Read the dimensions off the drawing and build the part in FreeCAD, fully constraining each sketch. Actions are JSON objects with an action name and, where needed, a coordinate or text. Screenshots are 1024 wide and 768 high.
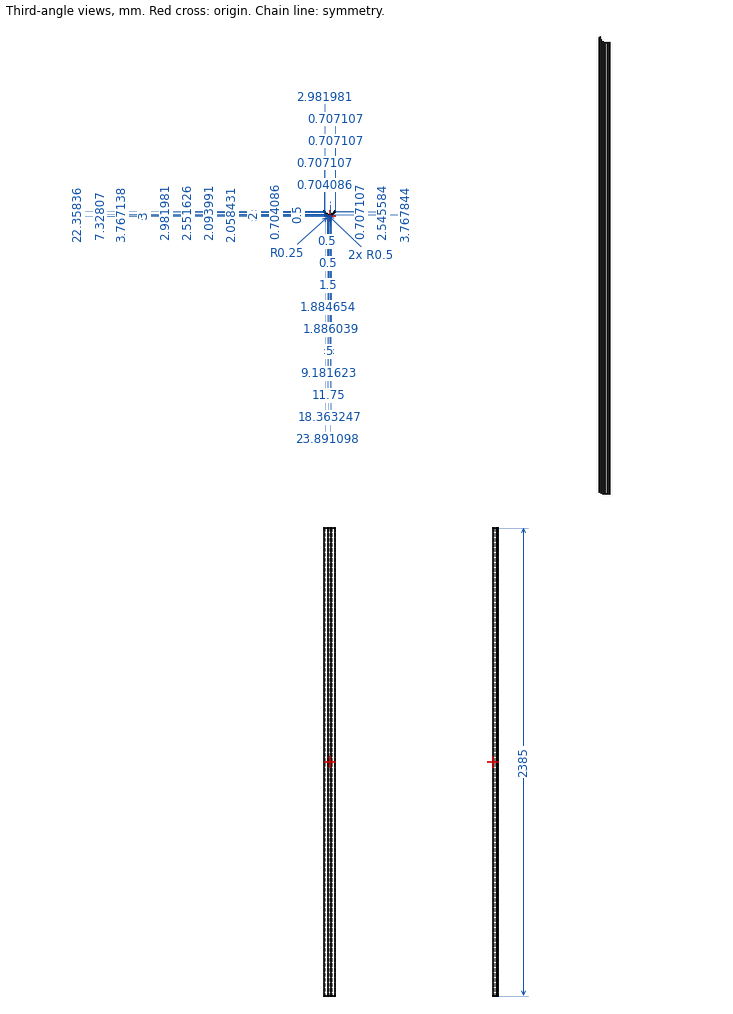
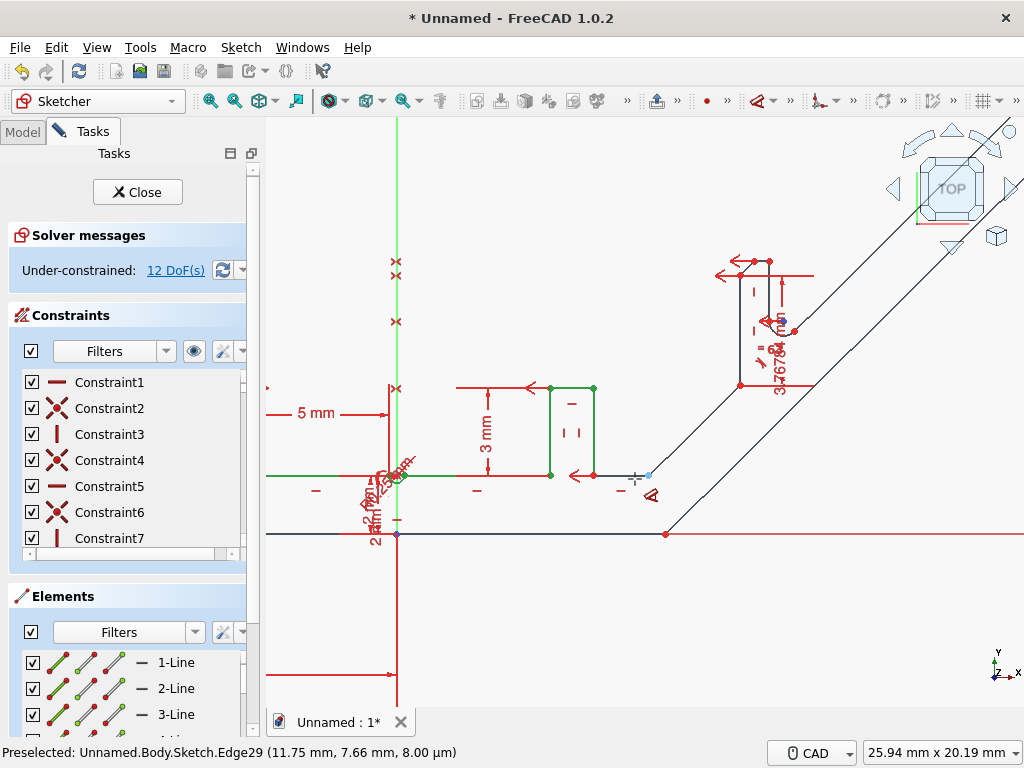
{"action": "left_click", "coordinate": [632, 476]}
{"action": "left_click", "coordinate": [621, 510]}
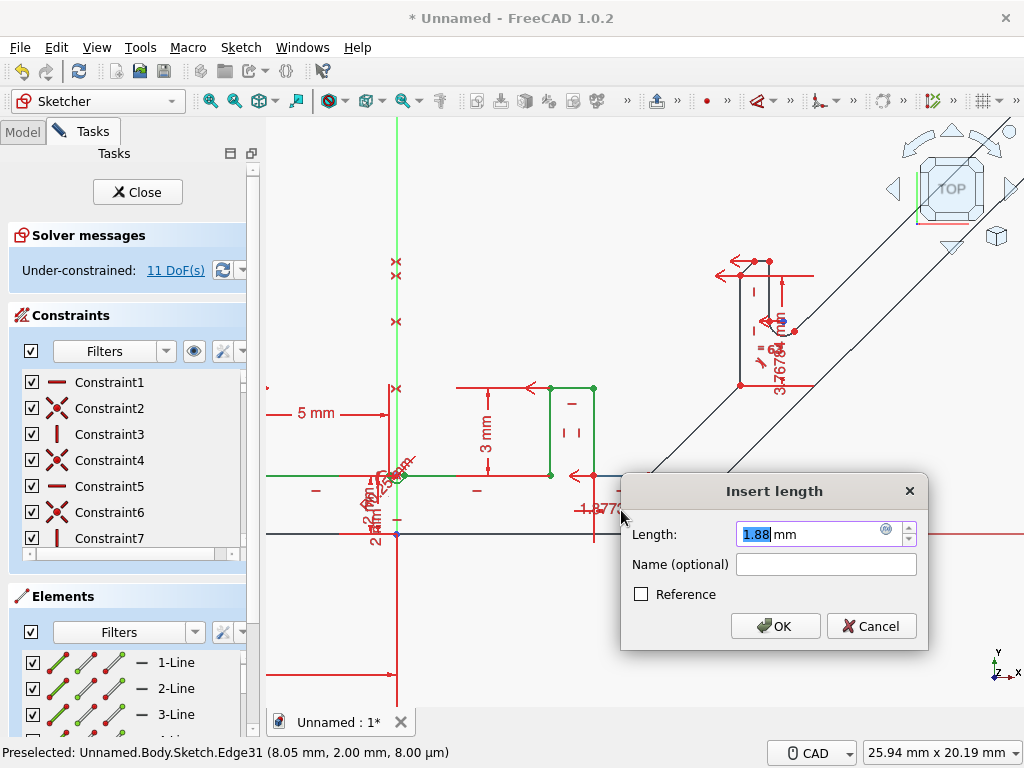
{"action": "type", "text": "1.886039"}
{"action": "key", "text": "Return"}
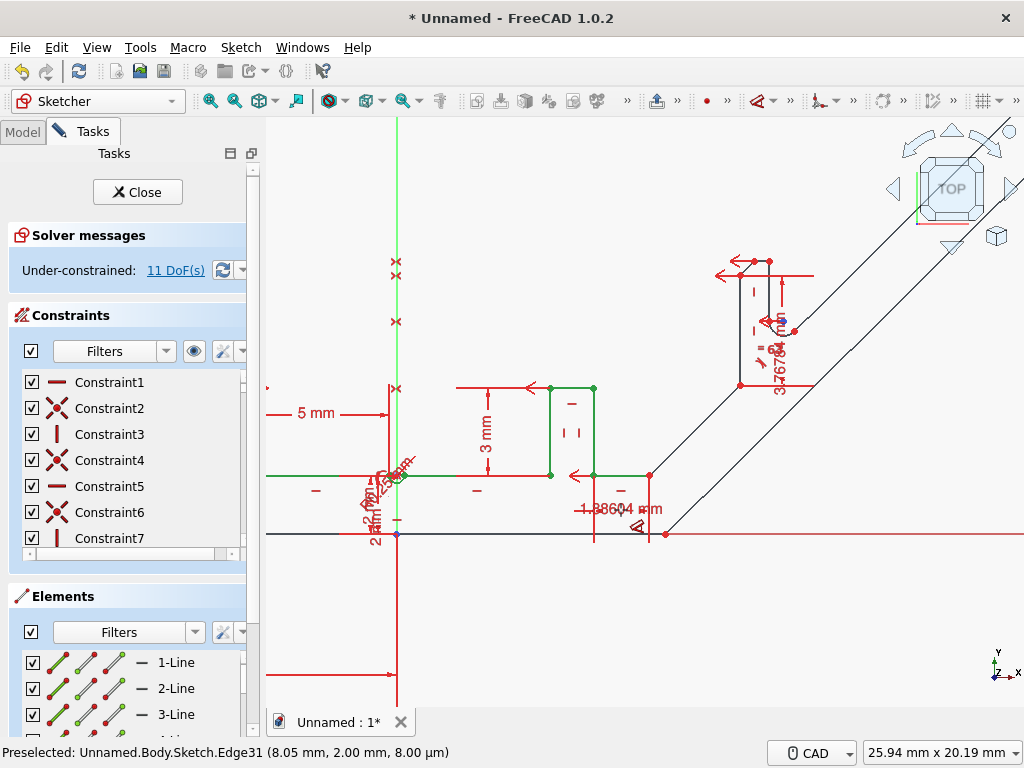
{"action": "scroll", "coordinate": [635, 479], "scroll_direction": "down", "scroll_amount": 7}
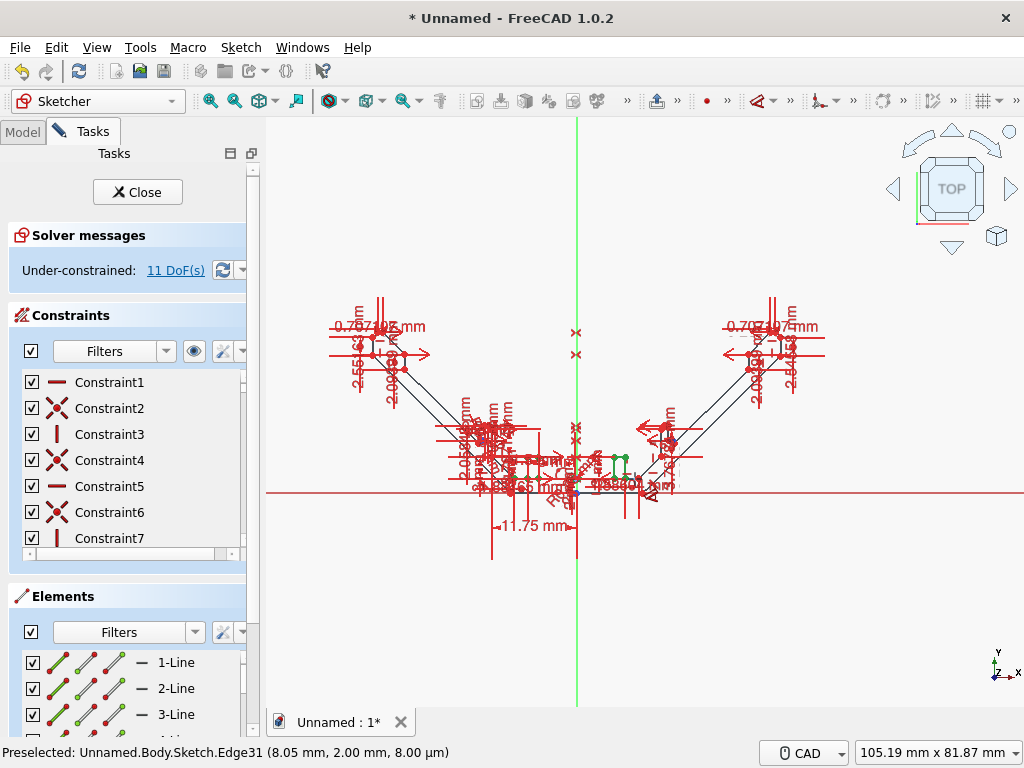
{"action": "scroll", "coordinate": [485, 441], "scroll_direction": "up", "scroll_amount": 7}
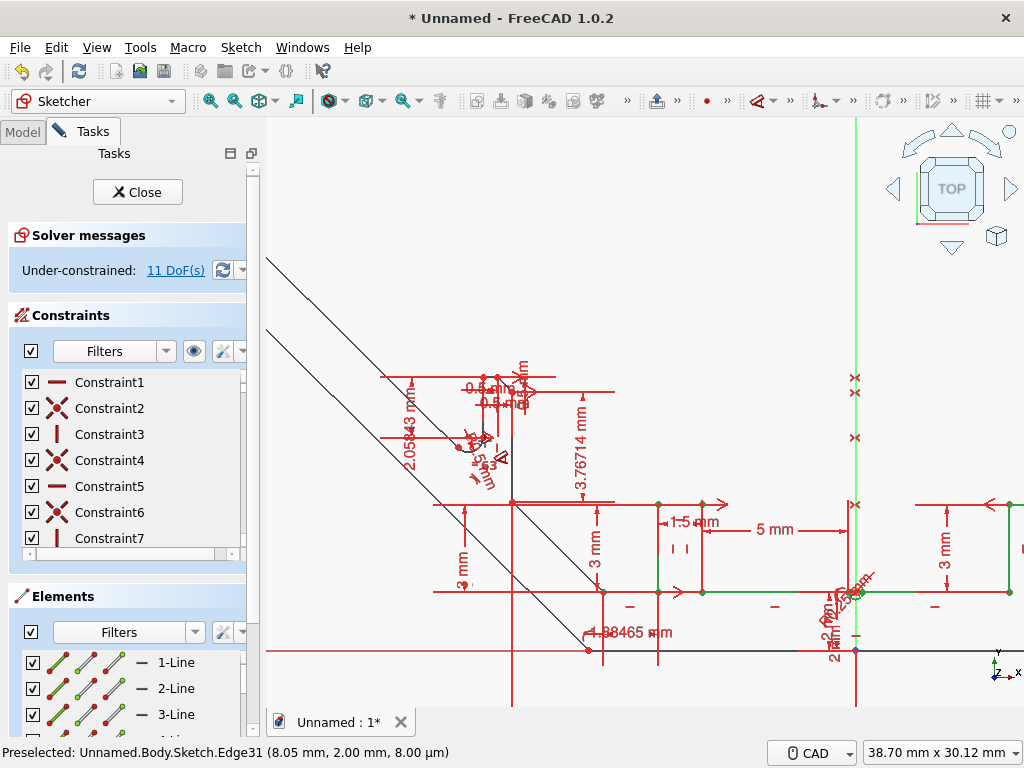
{"action": "left_click", "coordinate": [483, 438]}
{"action": "left_click", "coordinate": [449, 544]}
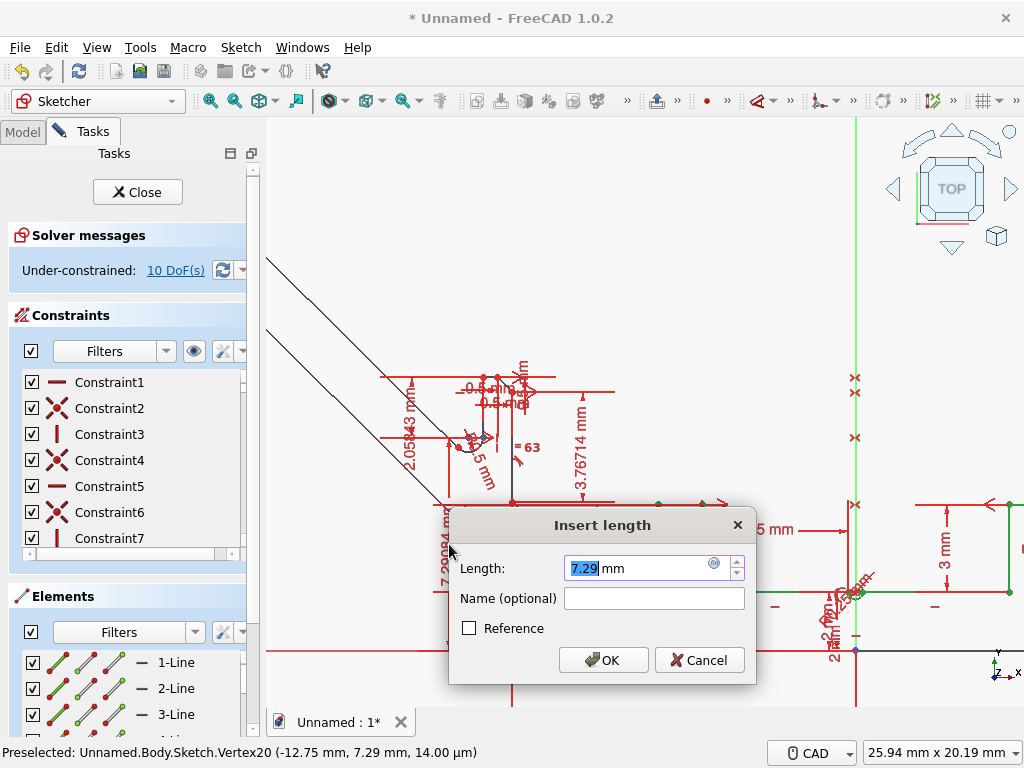
{"action": "type", "text": "7.32807"}
{"action": "key", "text": "Return"}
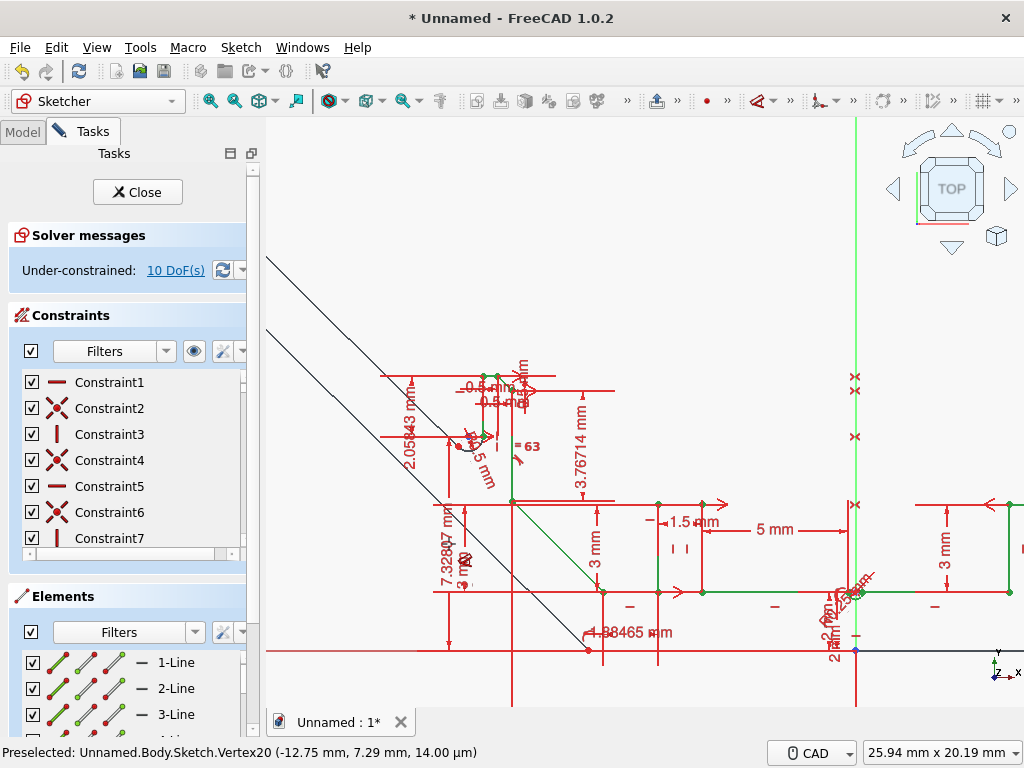
{"action": "scroll", "coordinate": [485, 441], "scroll_direction": "down", "scroll_amount": 7}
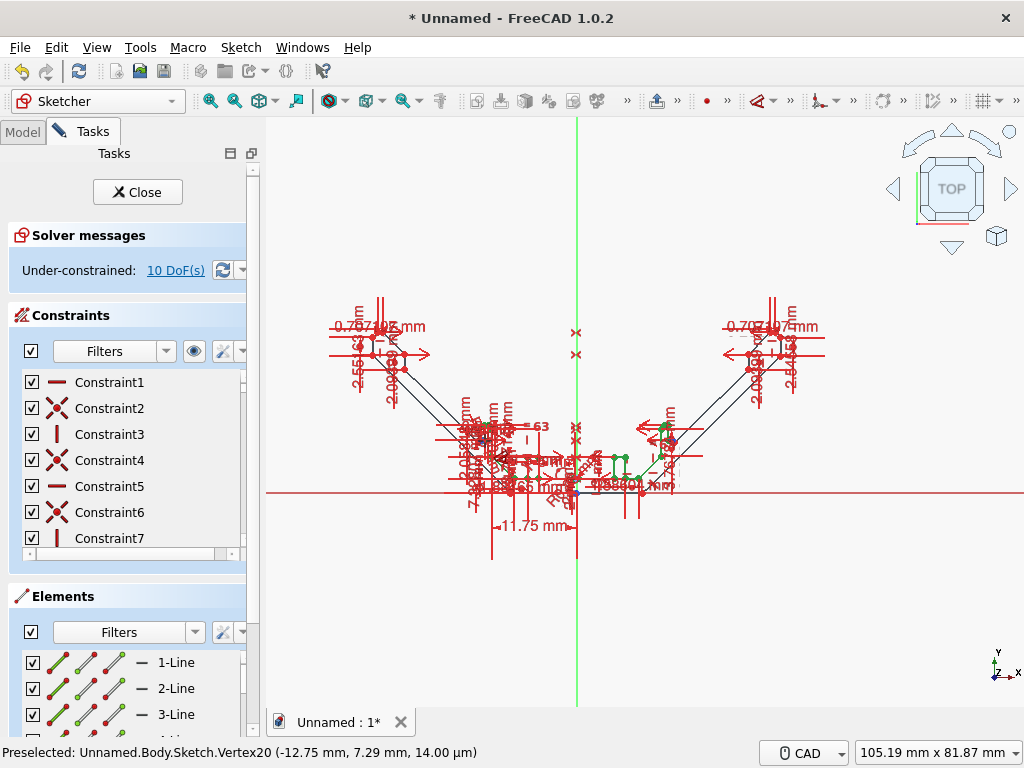
{"action": "left_click", "coordinate": [550, 493]}
{"action": "left_click", "coordinate": [607, 527]}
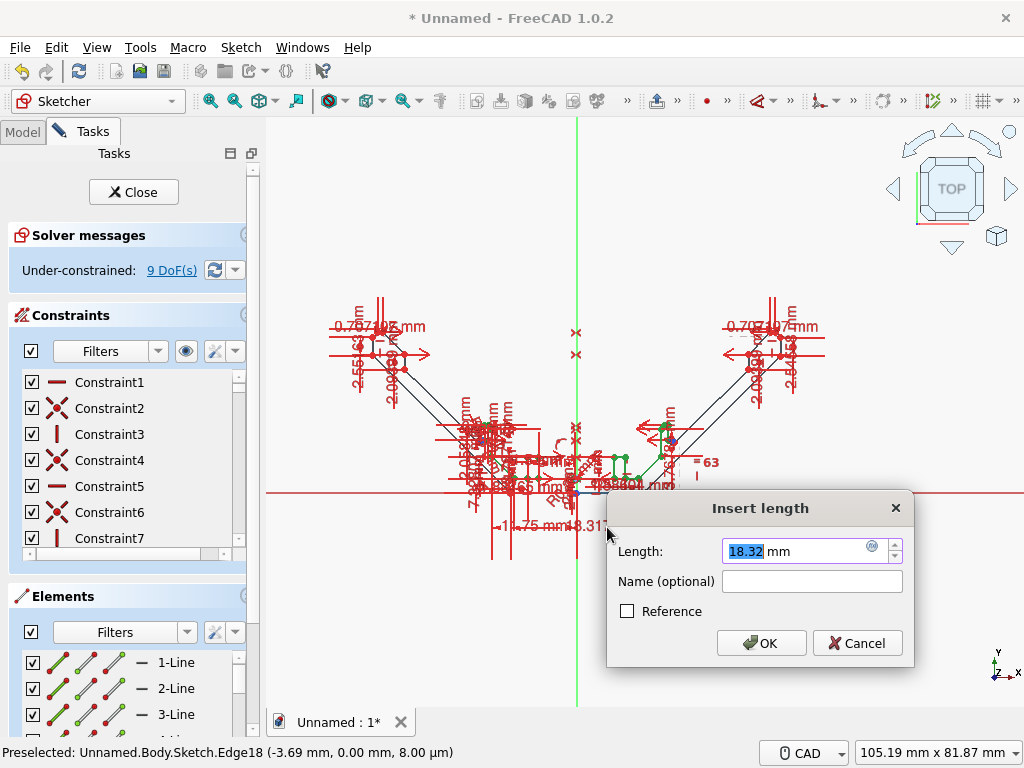
{"action": "type", "text": "18.363247"}
{"action": "key", "text": "Return"}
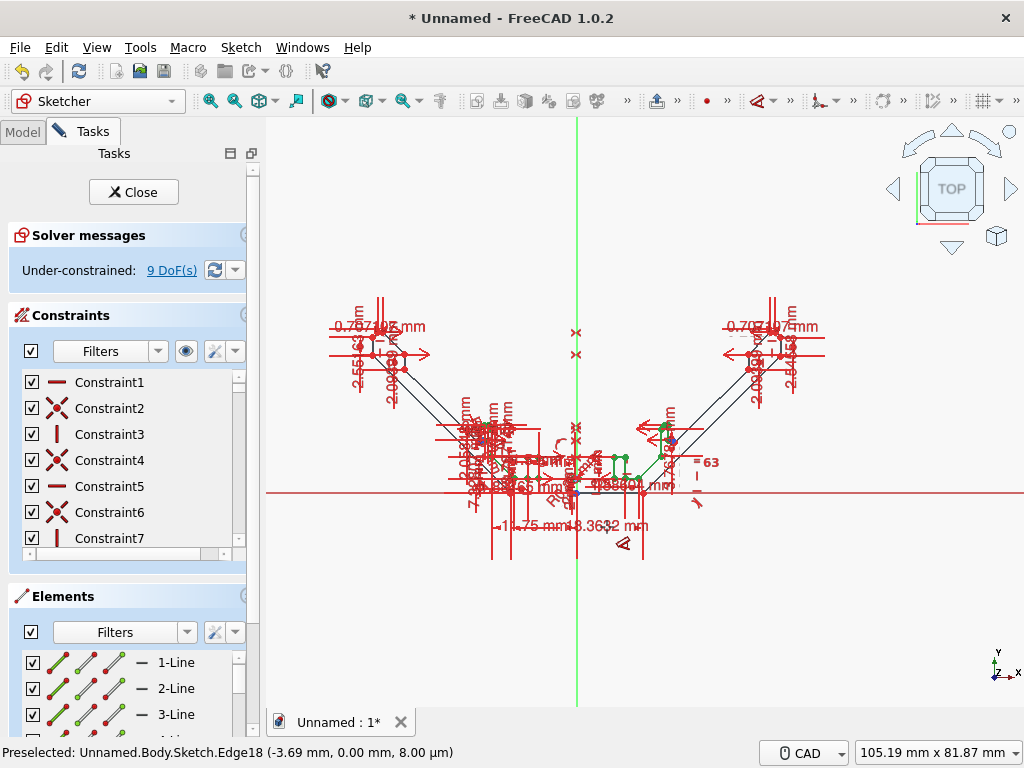
{"action": "scroll", "coordinate": [383, 332], "scroll_direction": "up", "scroll_amount": 5}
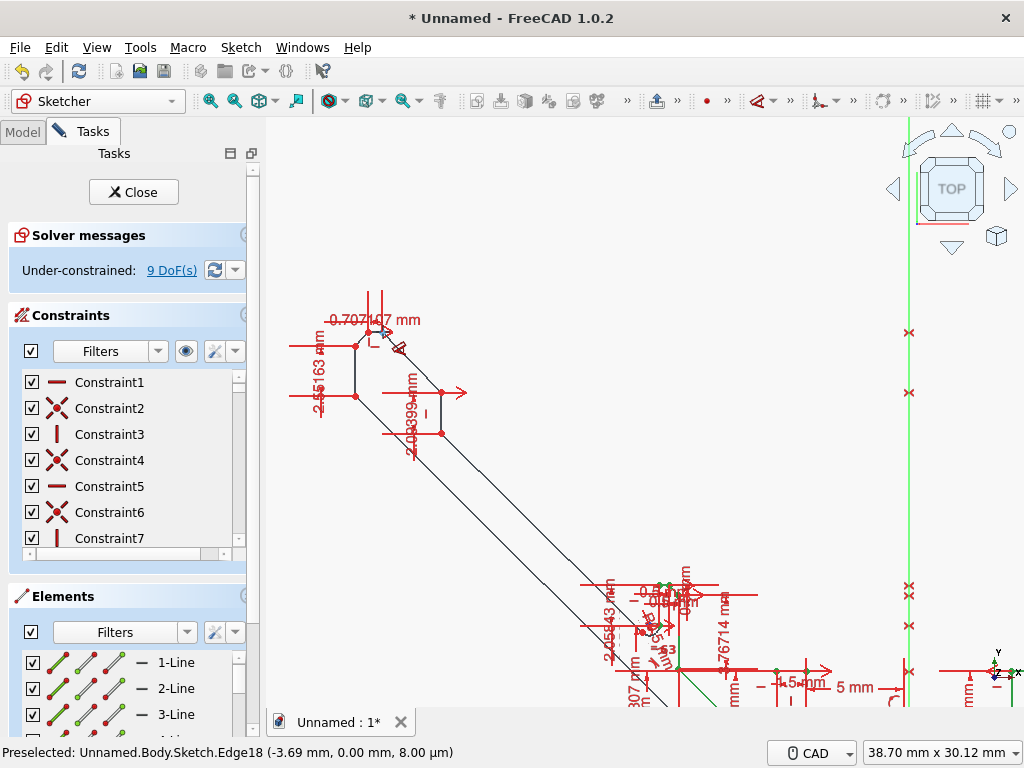
{"action": "left_click", "coordinate": [382, 332]}
{"action": "left_click", "coordinate": [348, 506]}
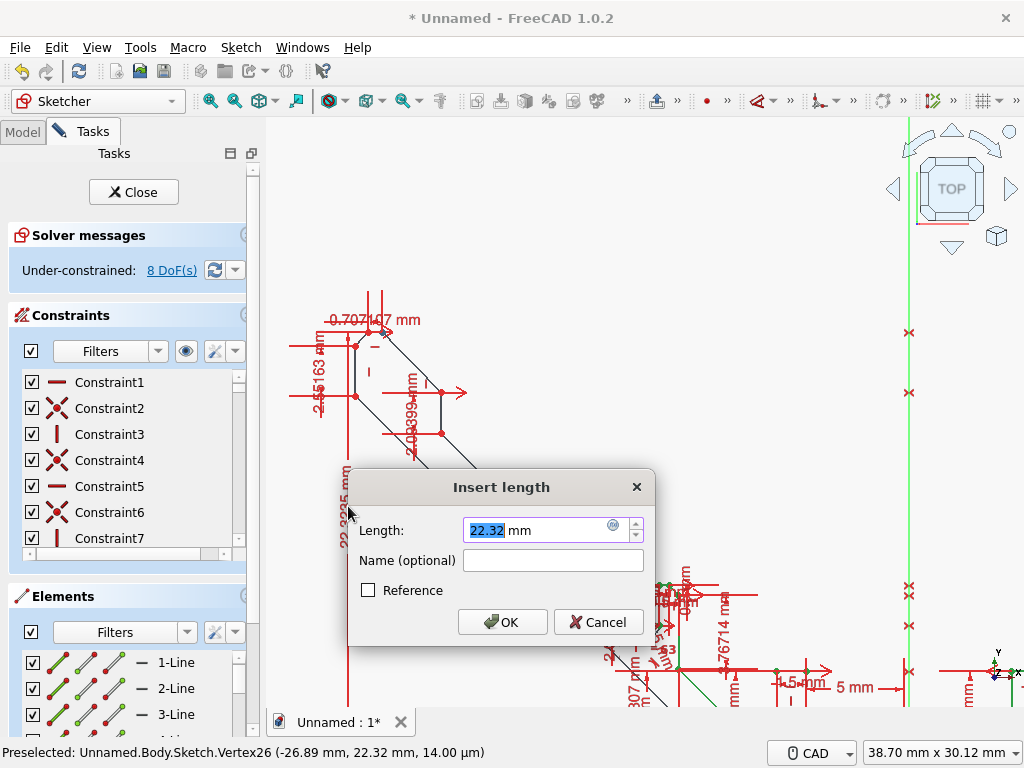
{"action": "type", "text": "22.35836"}
{"action": "key", "text": "Return"}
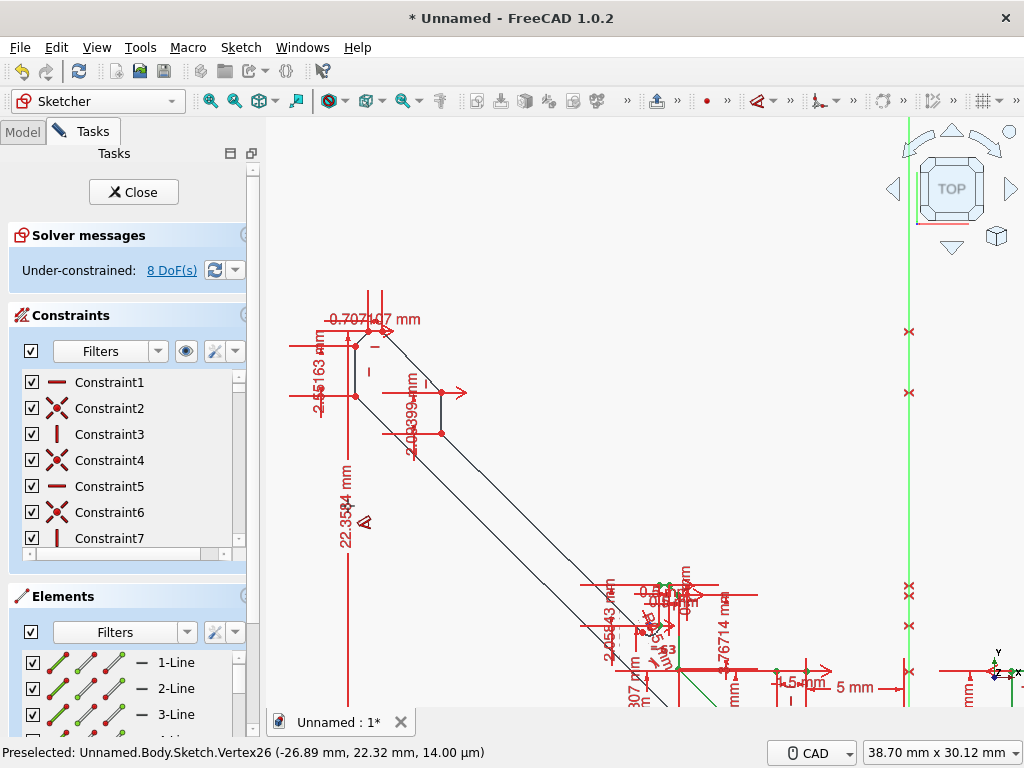
{"action": "scroll", "coordinate": [383, 331], "scroll_direction": "down", "scroll_amount": 5}